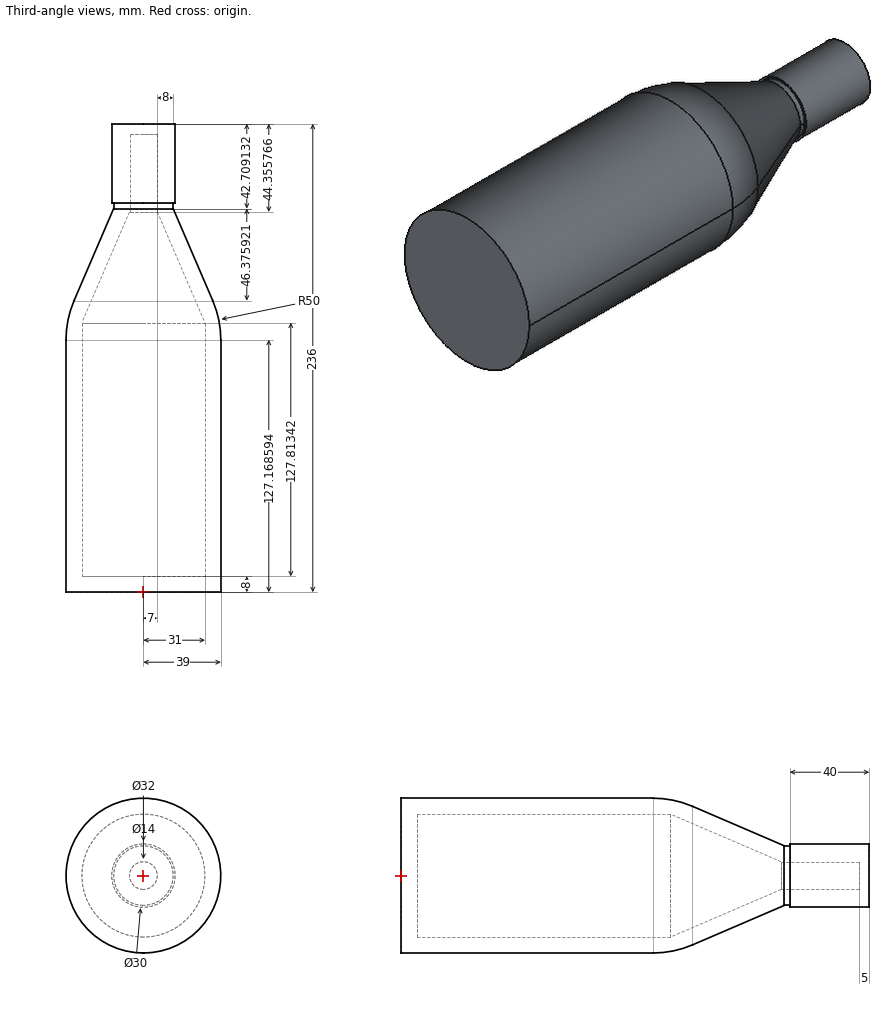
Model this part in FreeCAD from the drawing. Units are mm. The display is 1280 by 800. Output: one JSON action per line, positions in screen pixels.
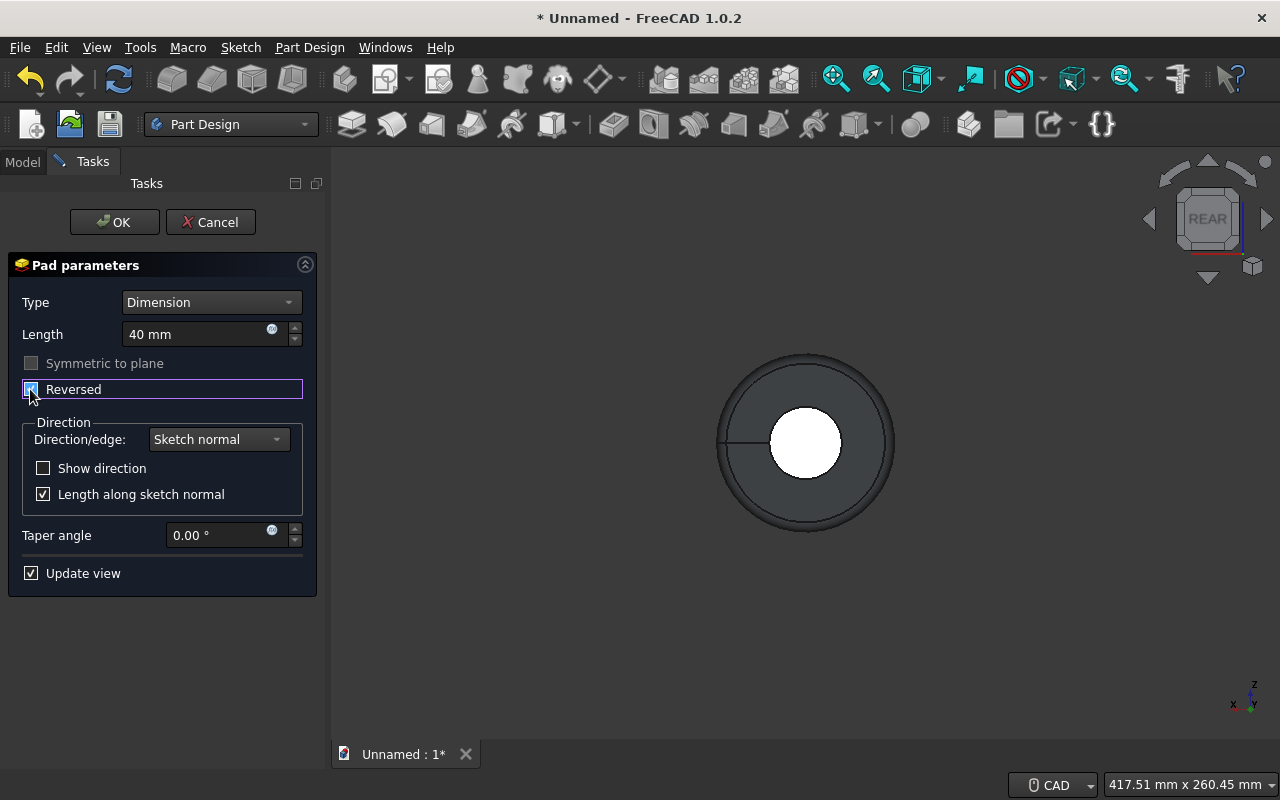
{"action": "left_click", "coordinate": [115, 222]}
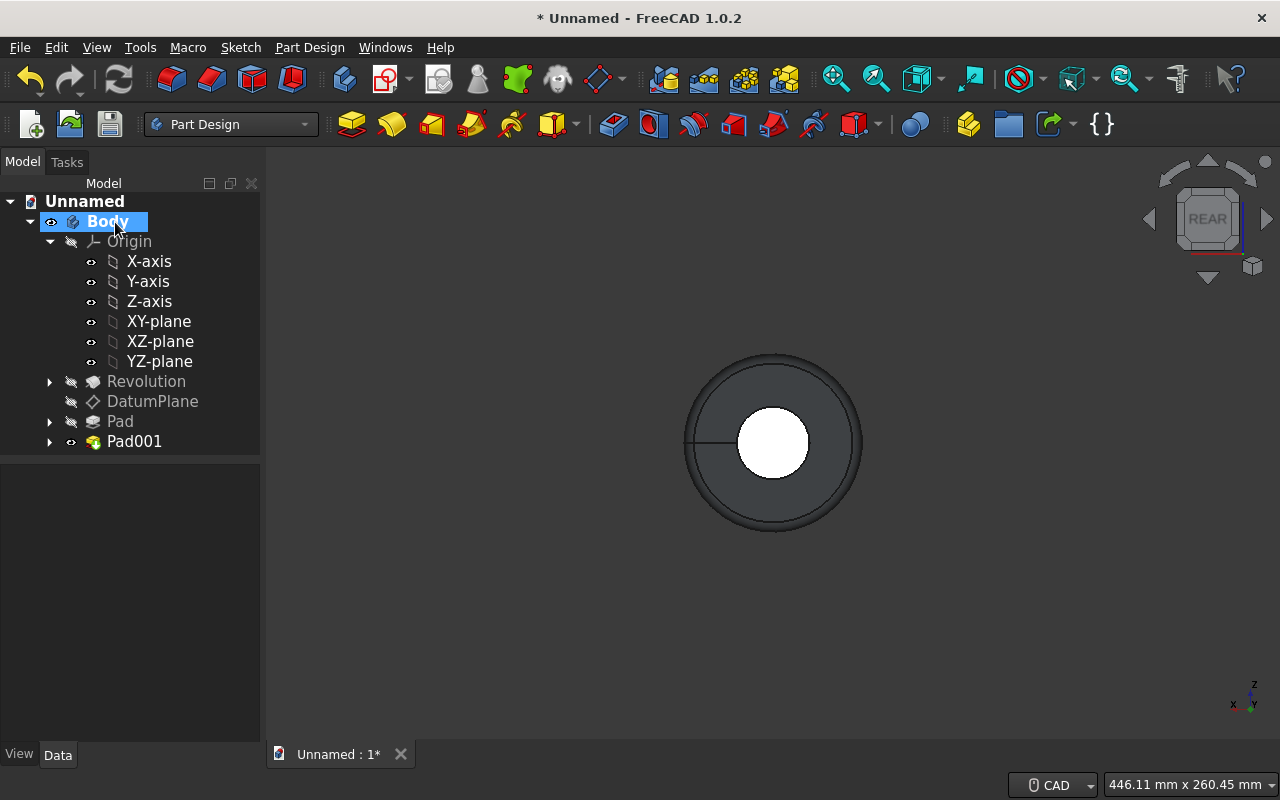
{"action": "key", "text": "0"}